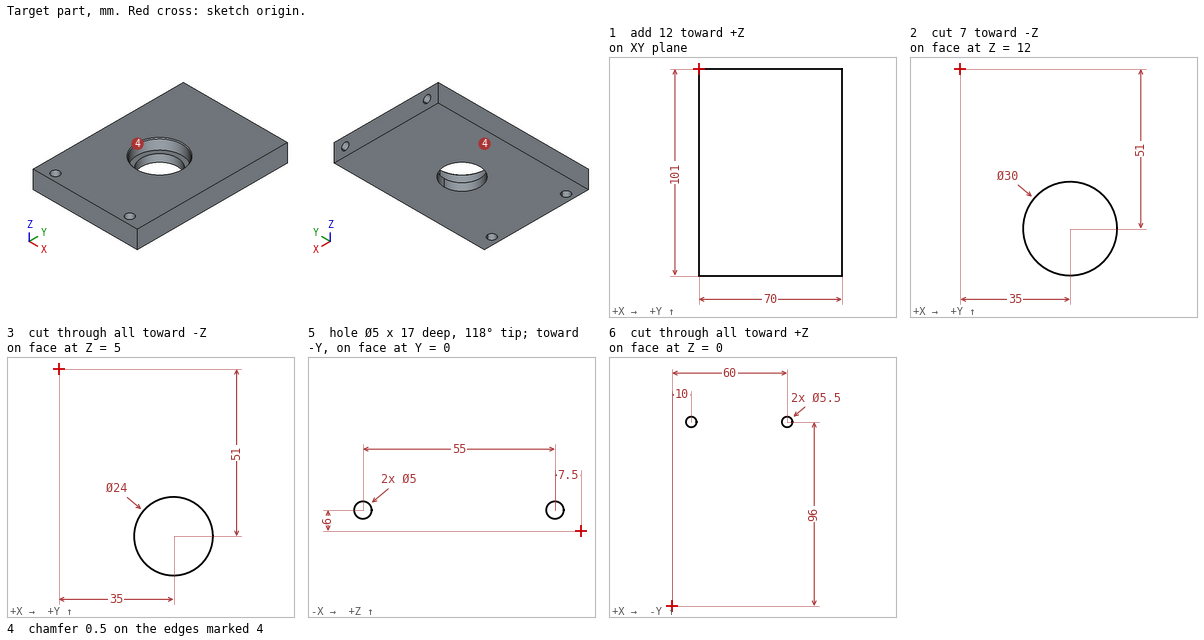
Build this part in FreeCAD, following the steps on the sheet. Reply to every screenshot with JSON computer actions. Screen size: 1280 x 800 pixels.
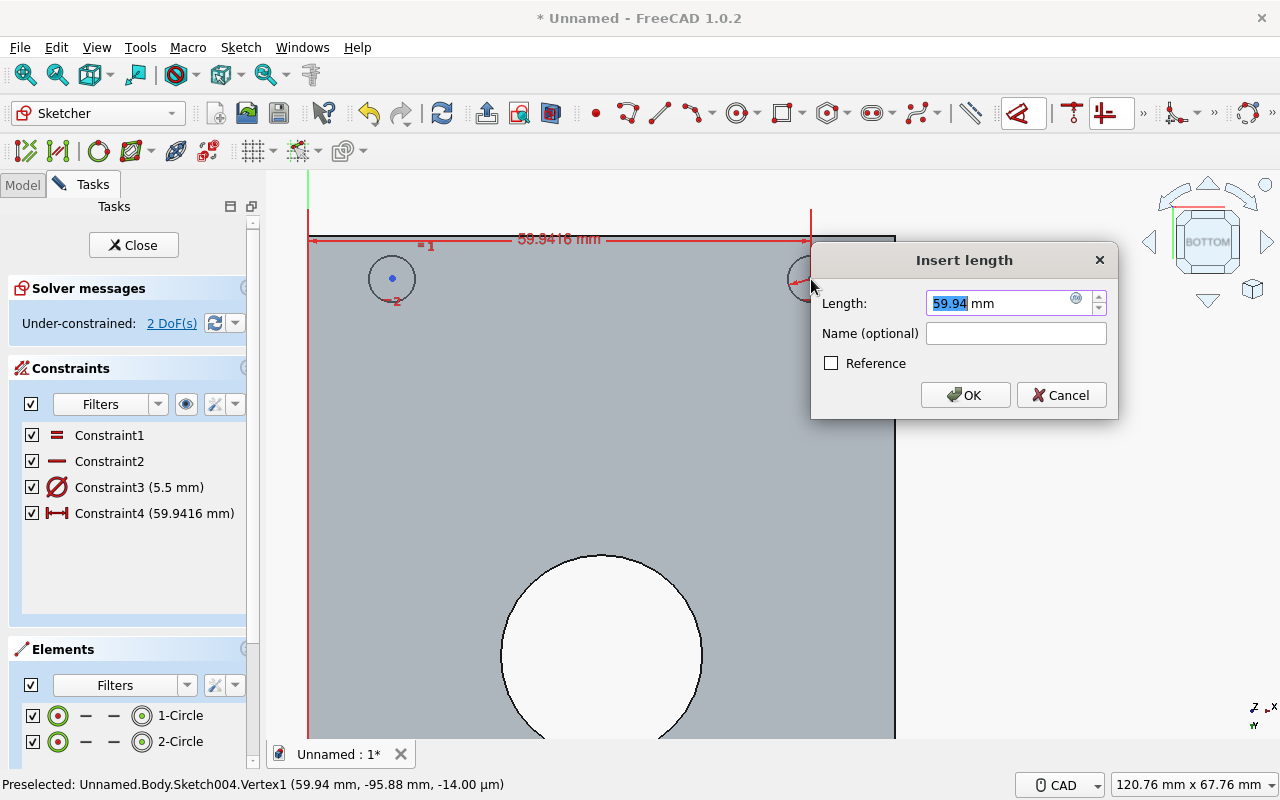
{"action": "type", "text": "60"}
{"action": "key", "text": "Return"}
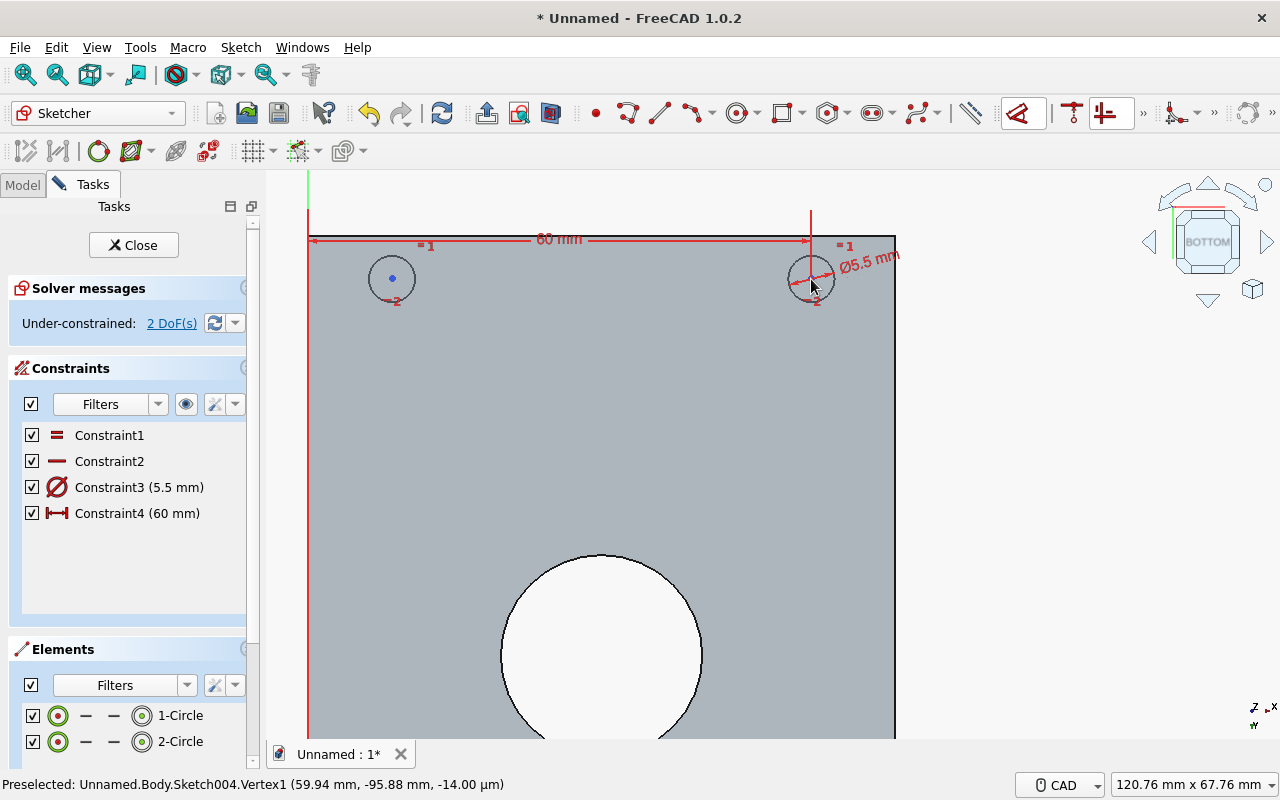
{"action": "left_click", "coordinate": [811, 279]}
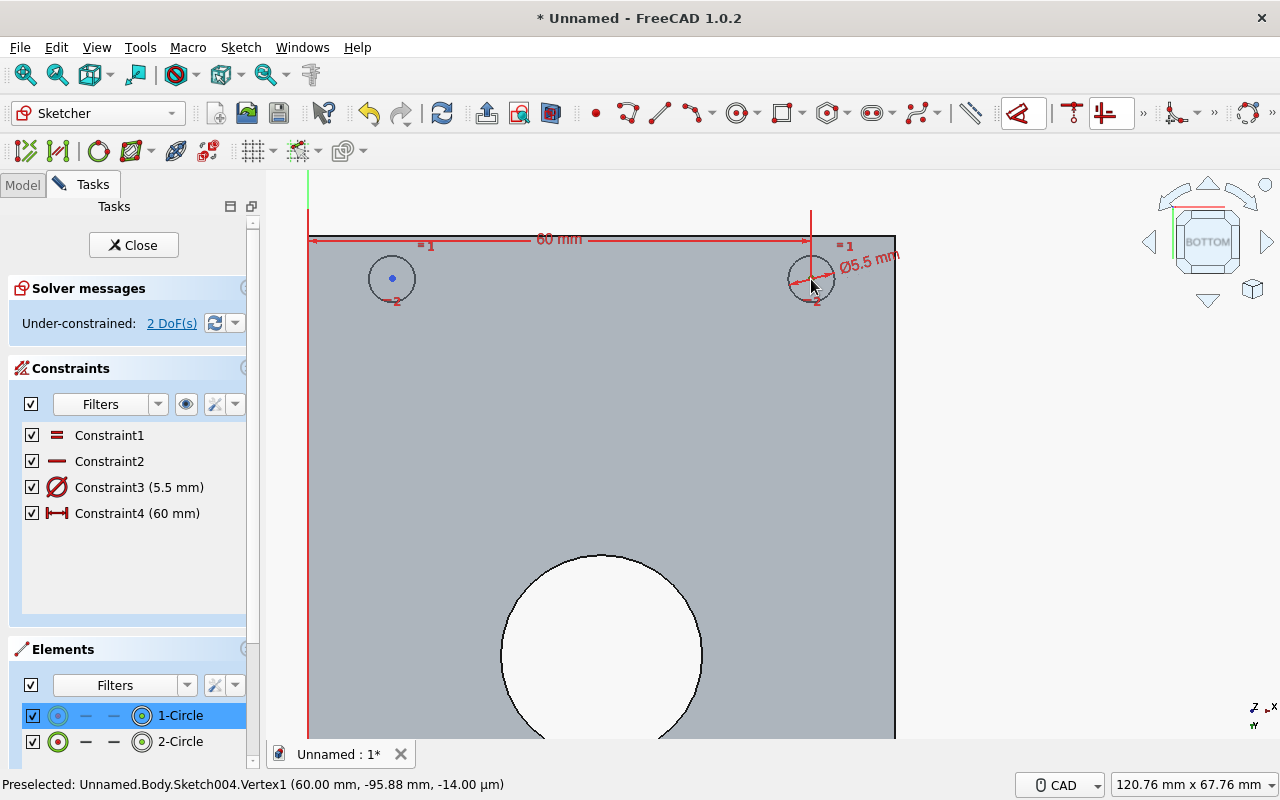
{"action": "left_click", "coordinate": [1040, 114]}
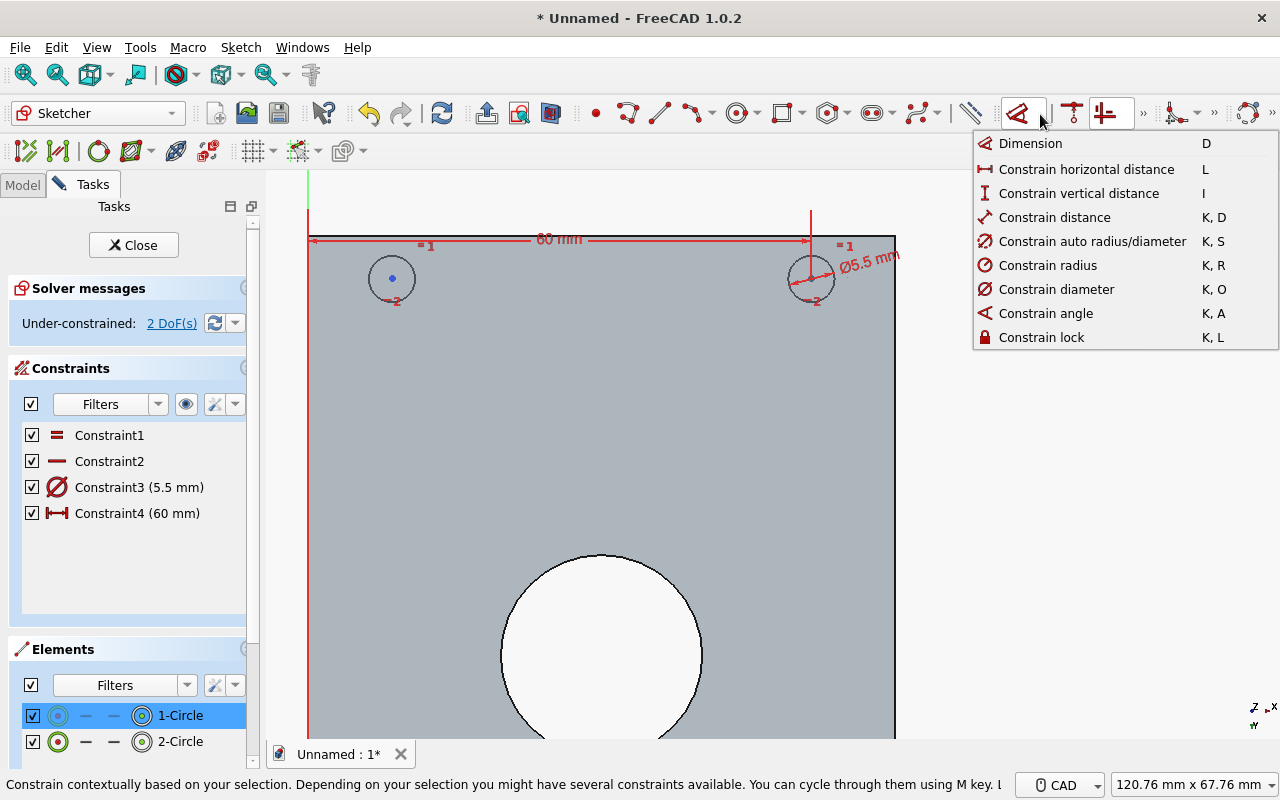
{"action": "left_click", "coordinate": [1126, 193]}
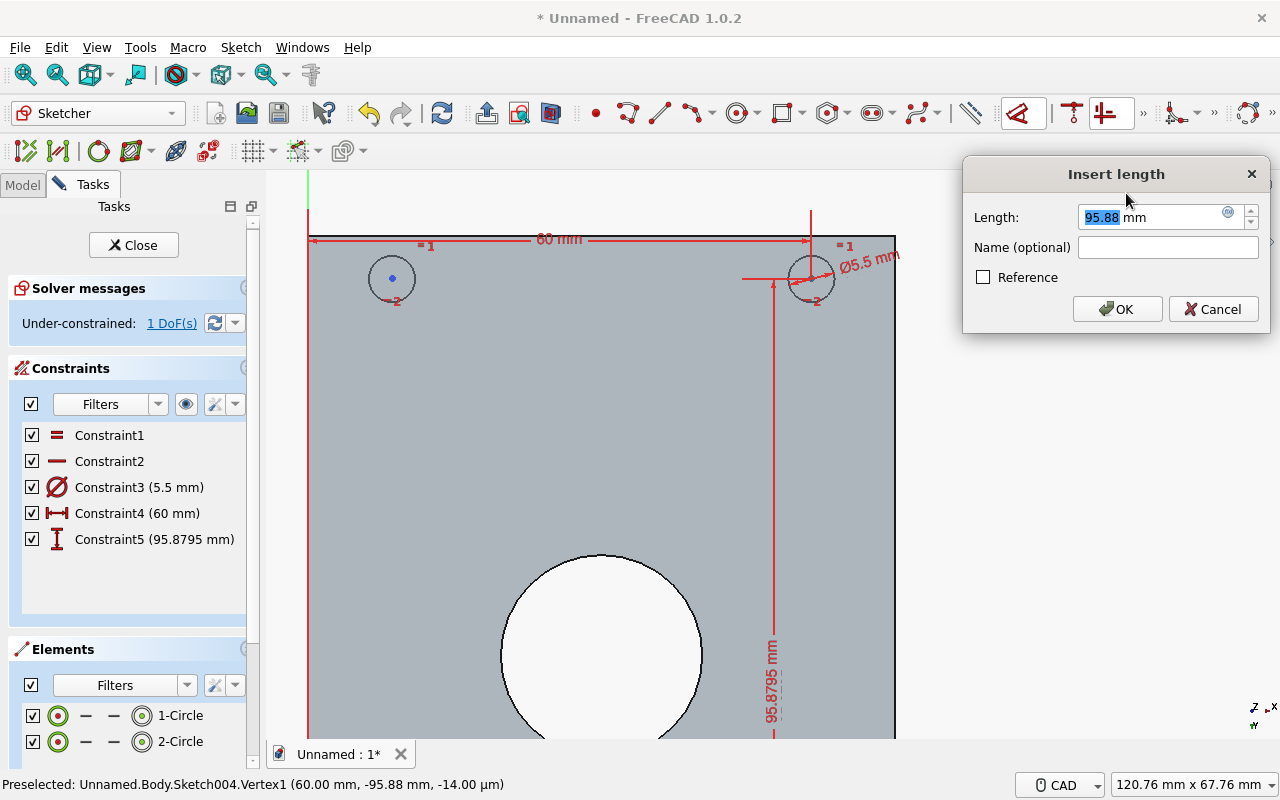
{"action": "type", "text": "96"}
{"action": "key", "text": "Return"}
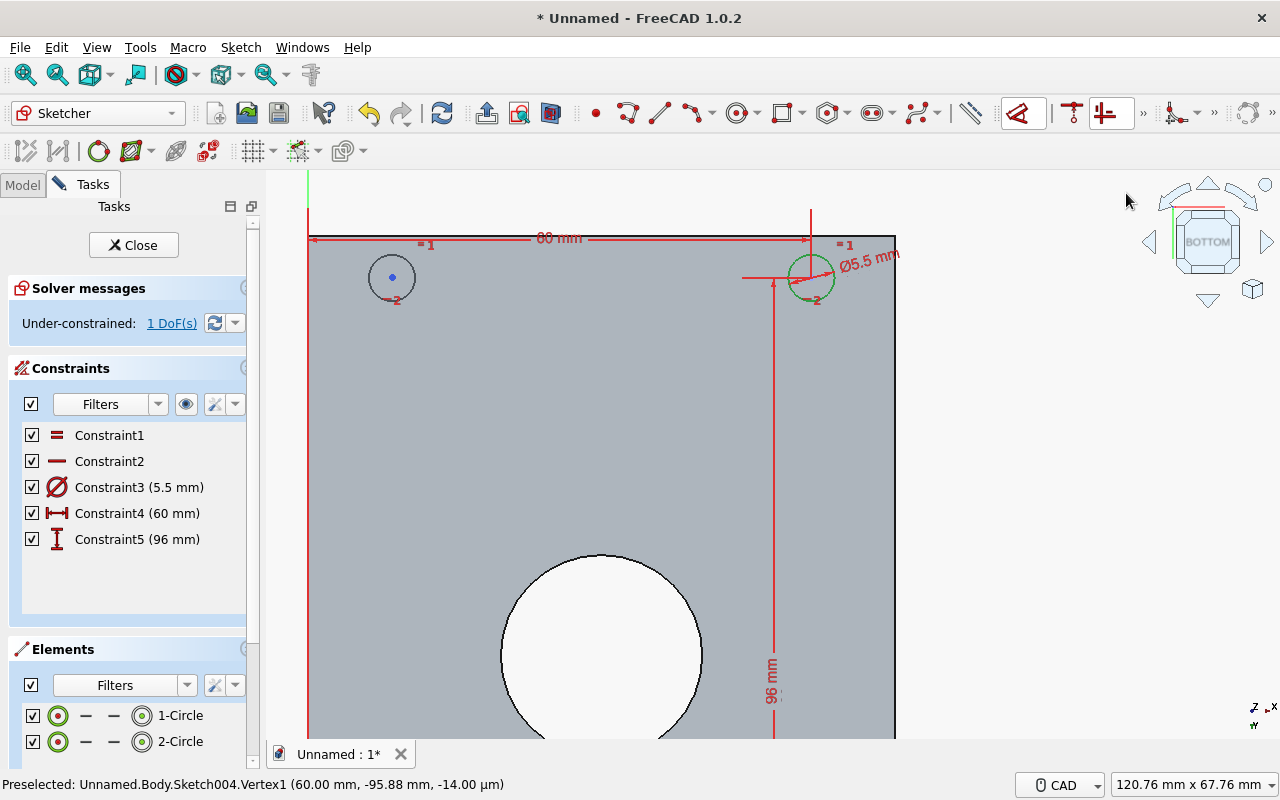
{"action": "left_click", "coordinate": [392, 278]}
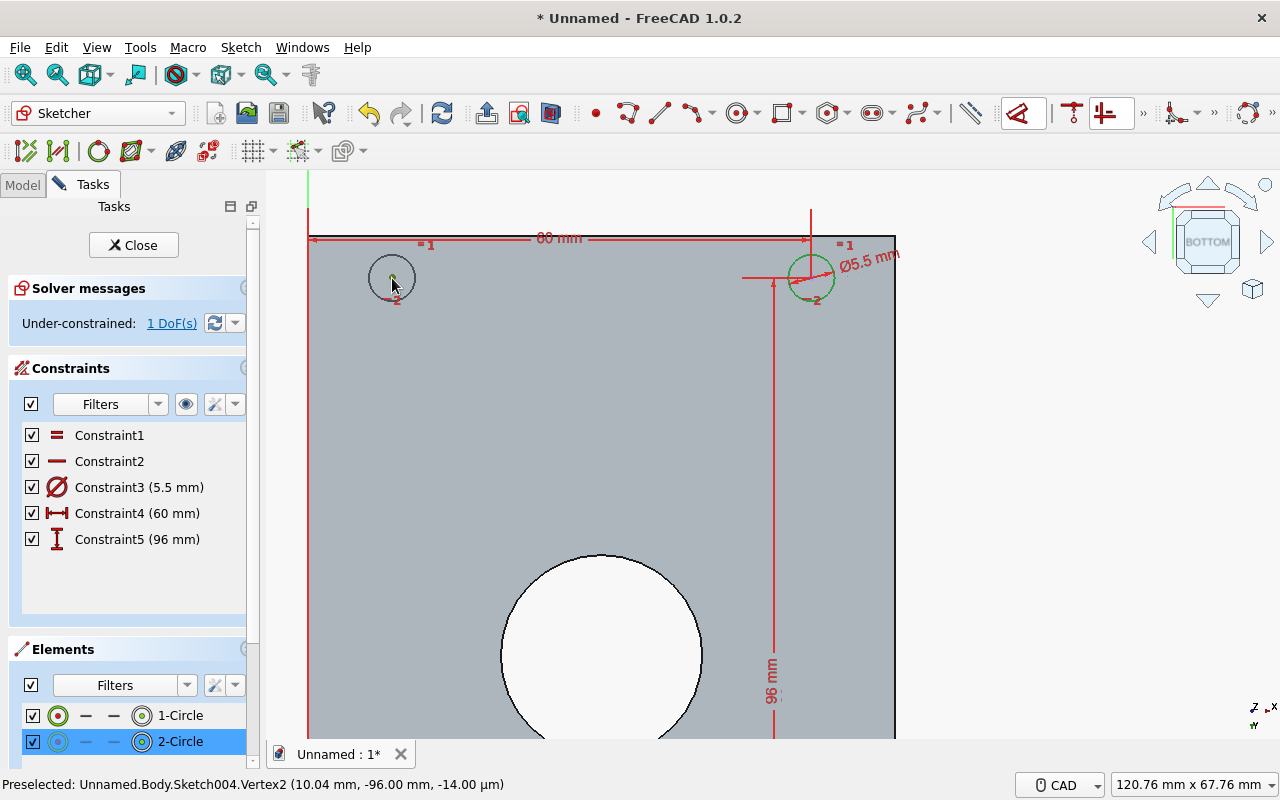
{"action": "left_click", "coordinate": [1040, 114]}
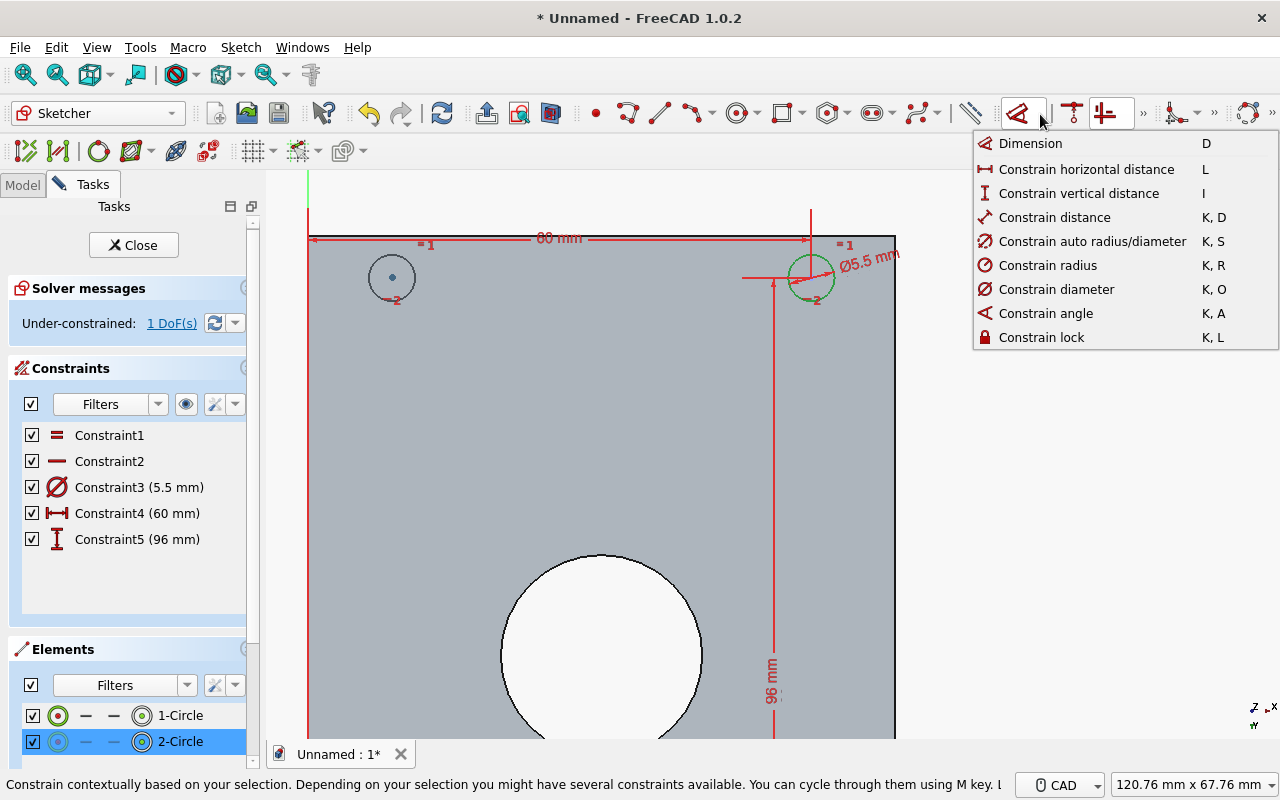
{"action": "left_click", "coordinate": [1126, 169]}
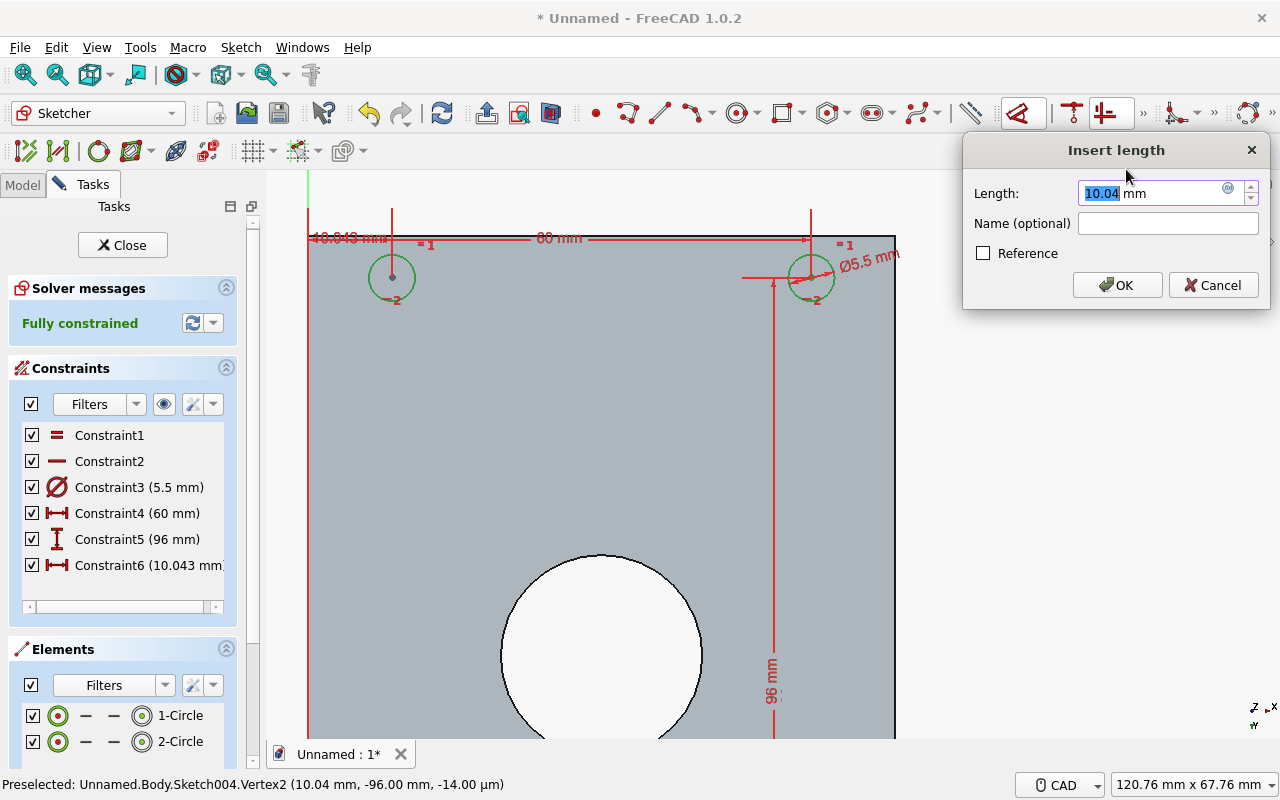
{"action": "type", "text": "10"}
{"action": "key", "text": "Return"}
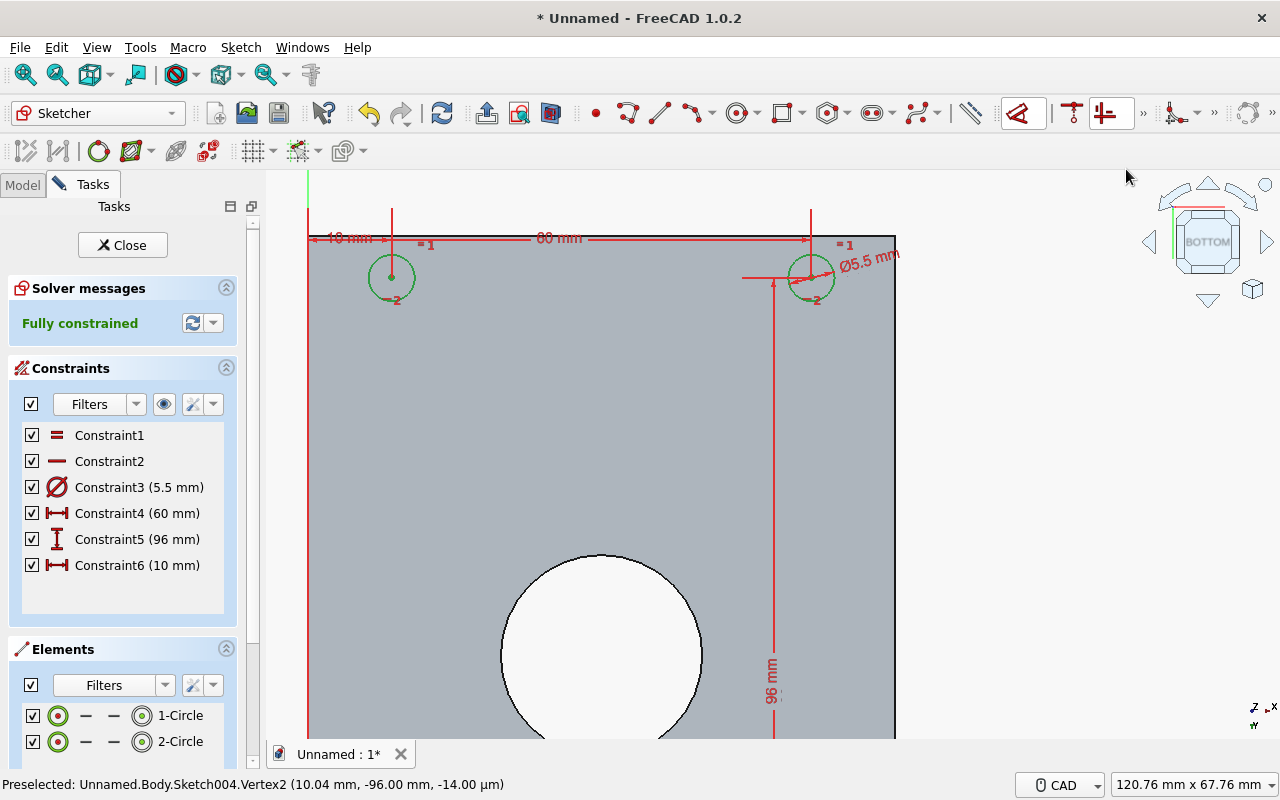
{"action": "left_click", "coordinate": [123, 245]}